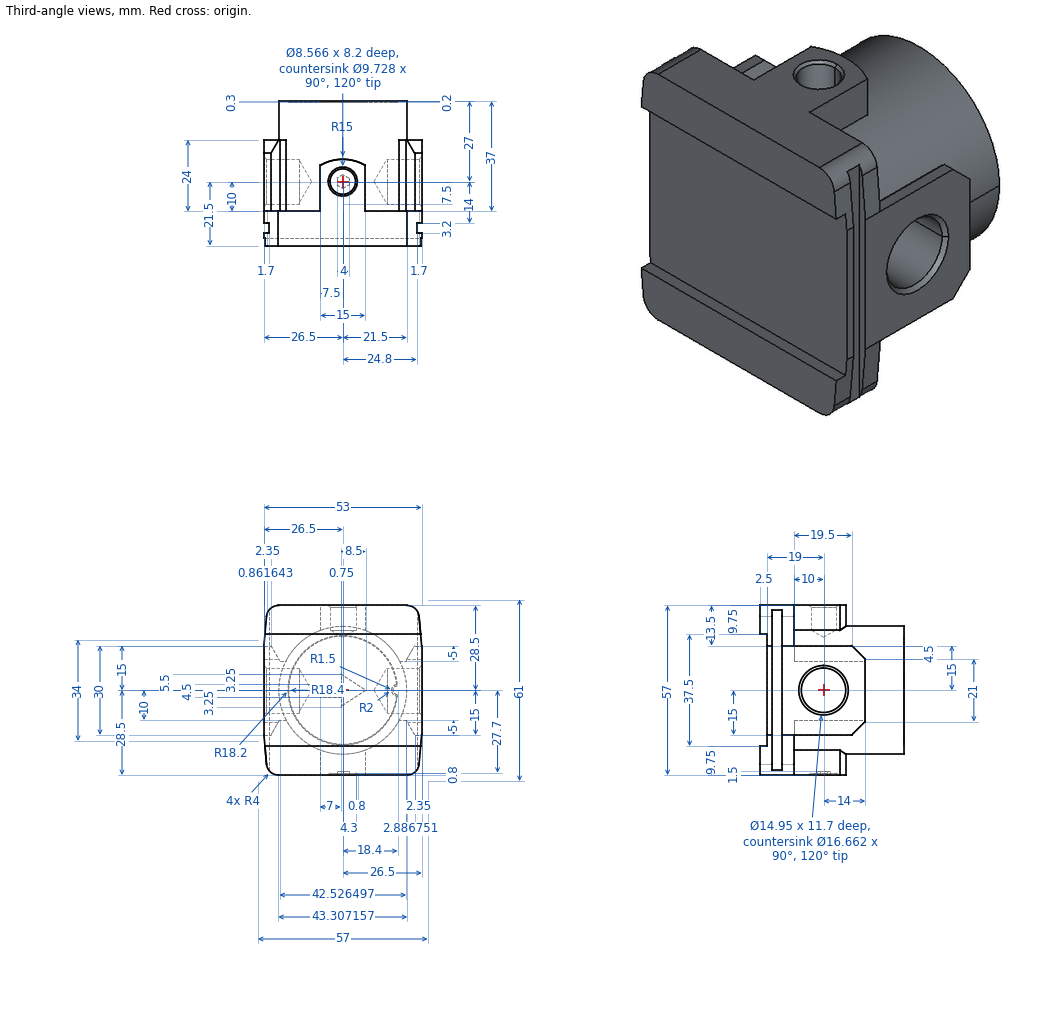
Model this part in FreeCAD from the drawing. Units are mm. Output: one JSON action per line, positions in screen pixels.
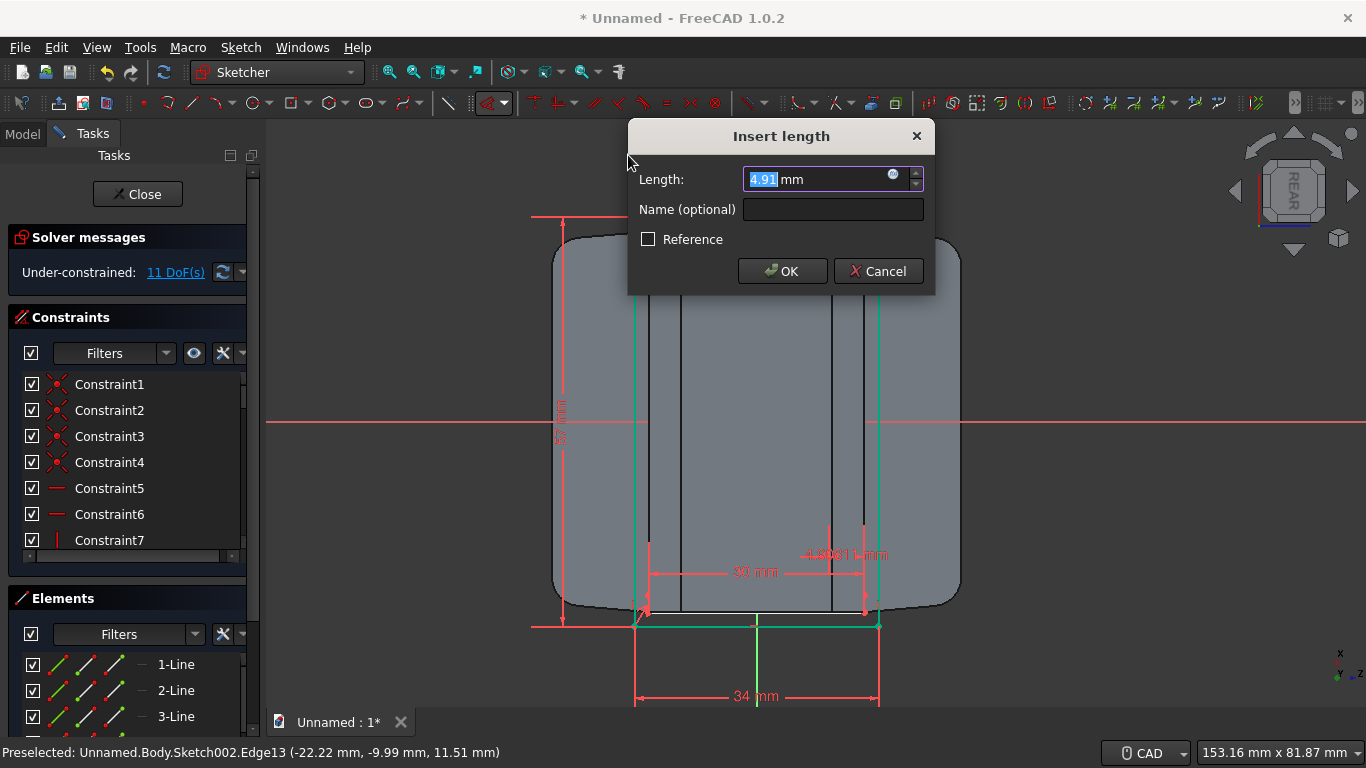
{"action": "type", "text": "5"}
{"action": "key", "text": "Return"}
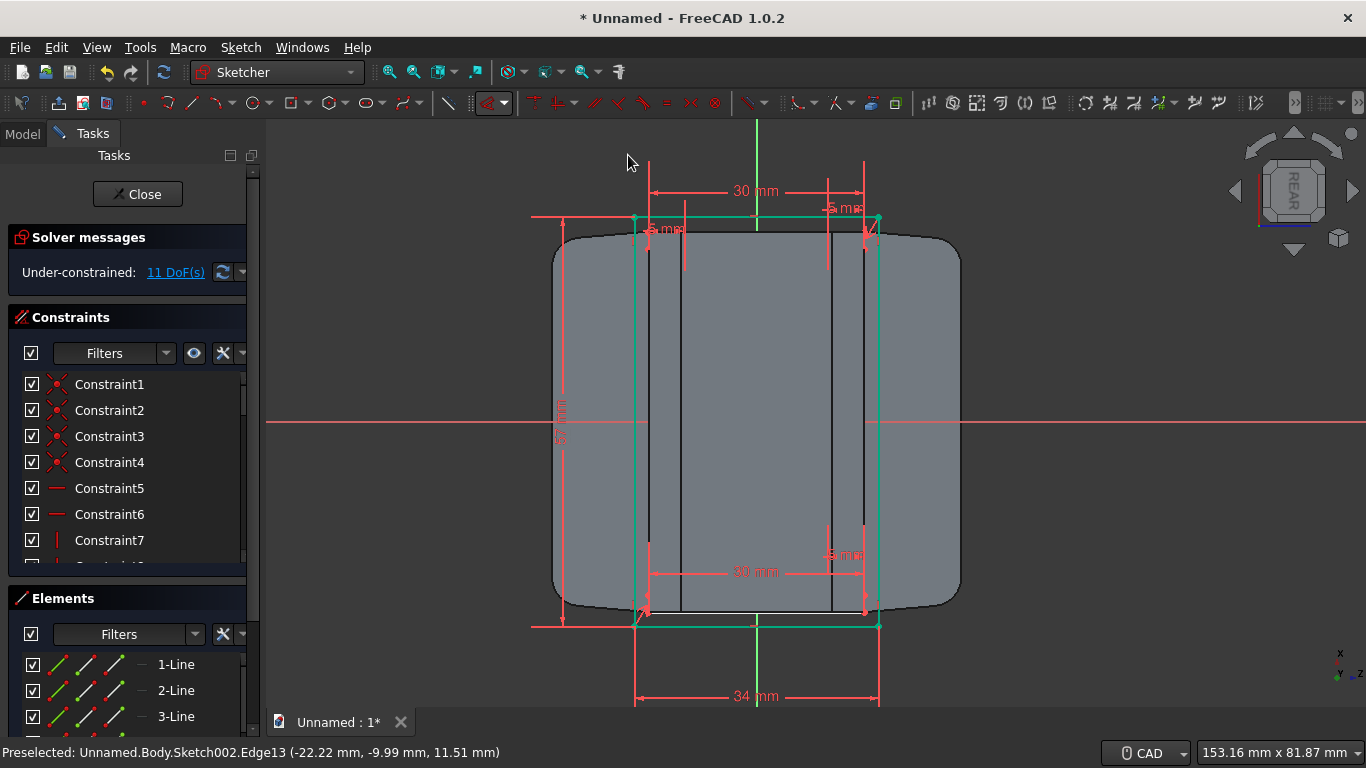
{"action": "left_click", "coordinate": [685, 576]}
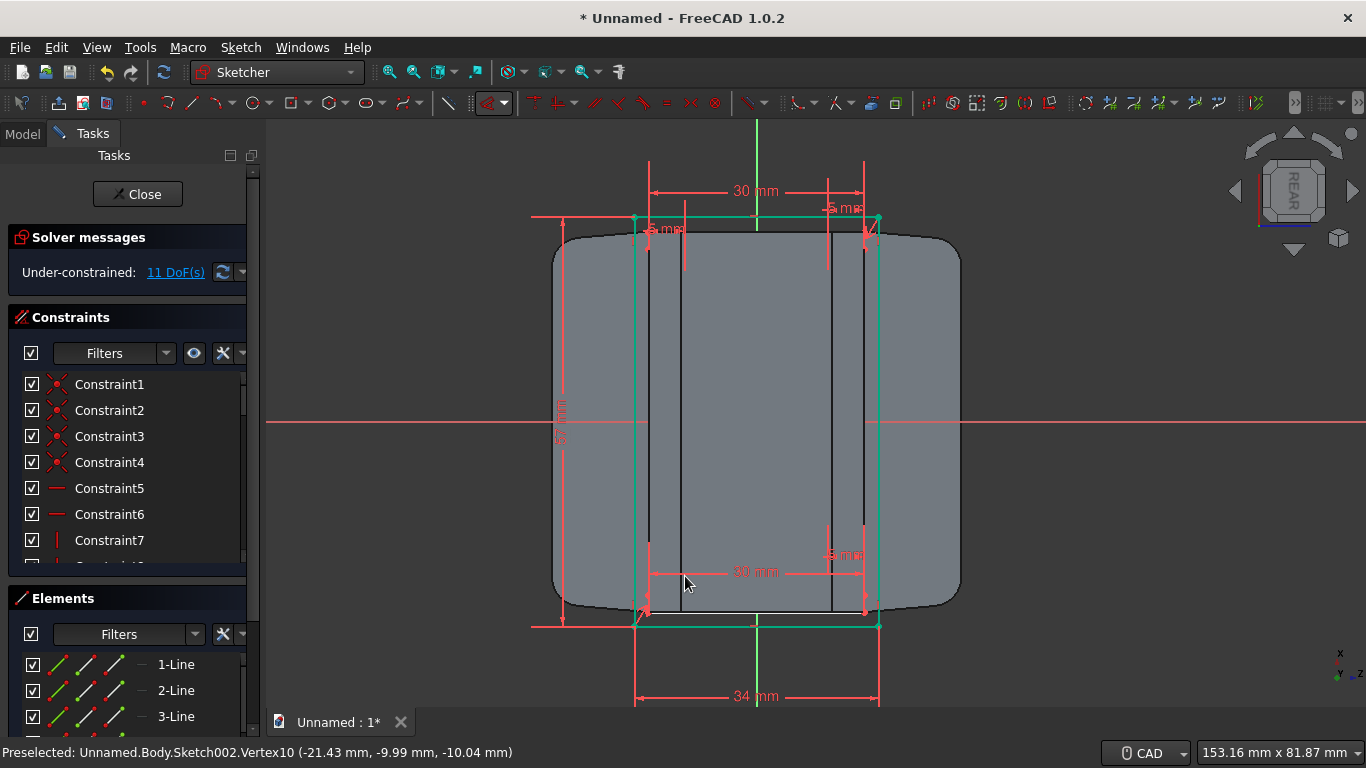
{"action": "left_click", "coordinate": [506, 104]}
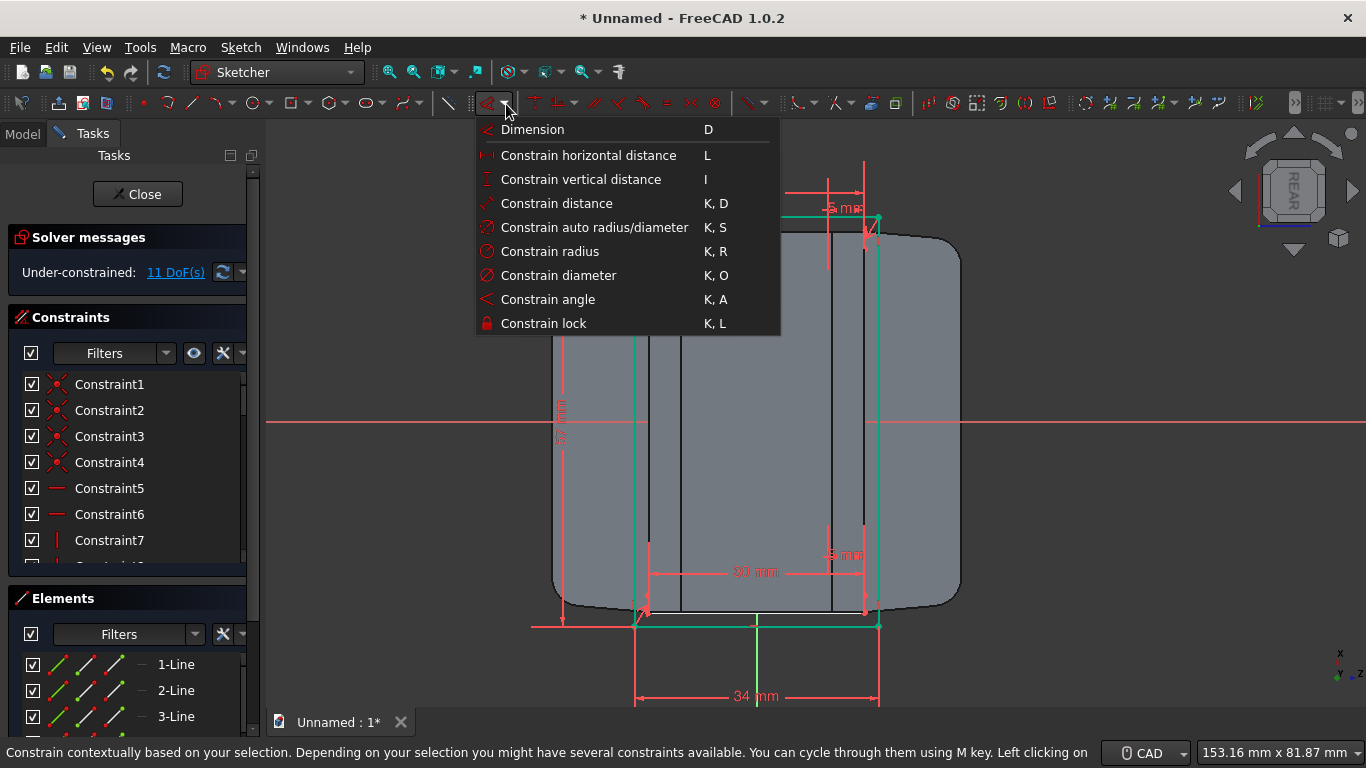
{"action": "left_click", "coordinate": [628, 155]}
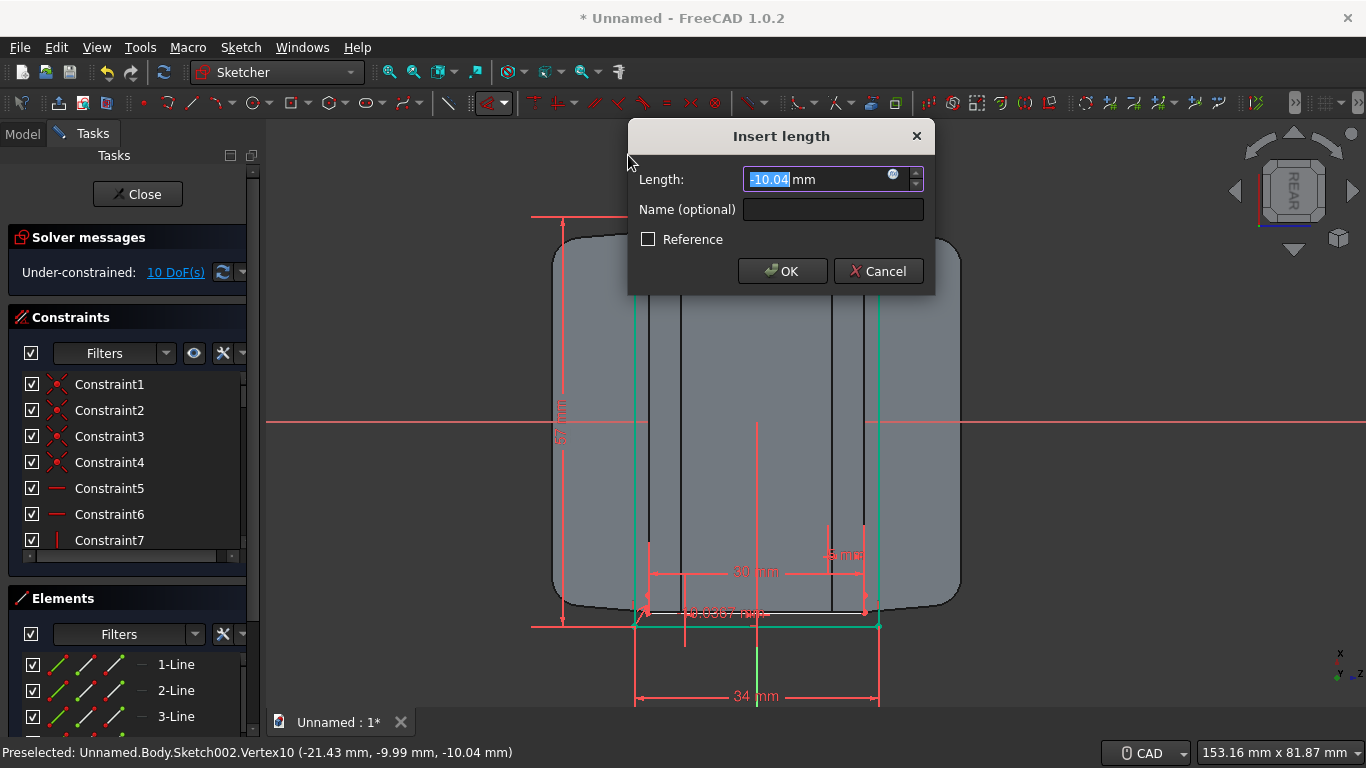
{"action": "type", "text": "-10"}
{"action": "key", "text": "Return"}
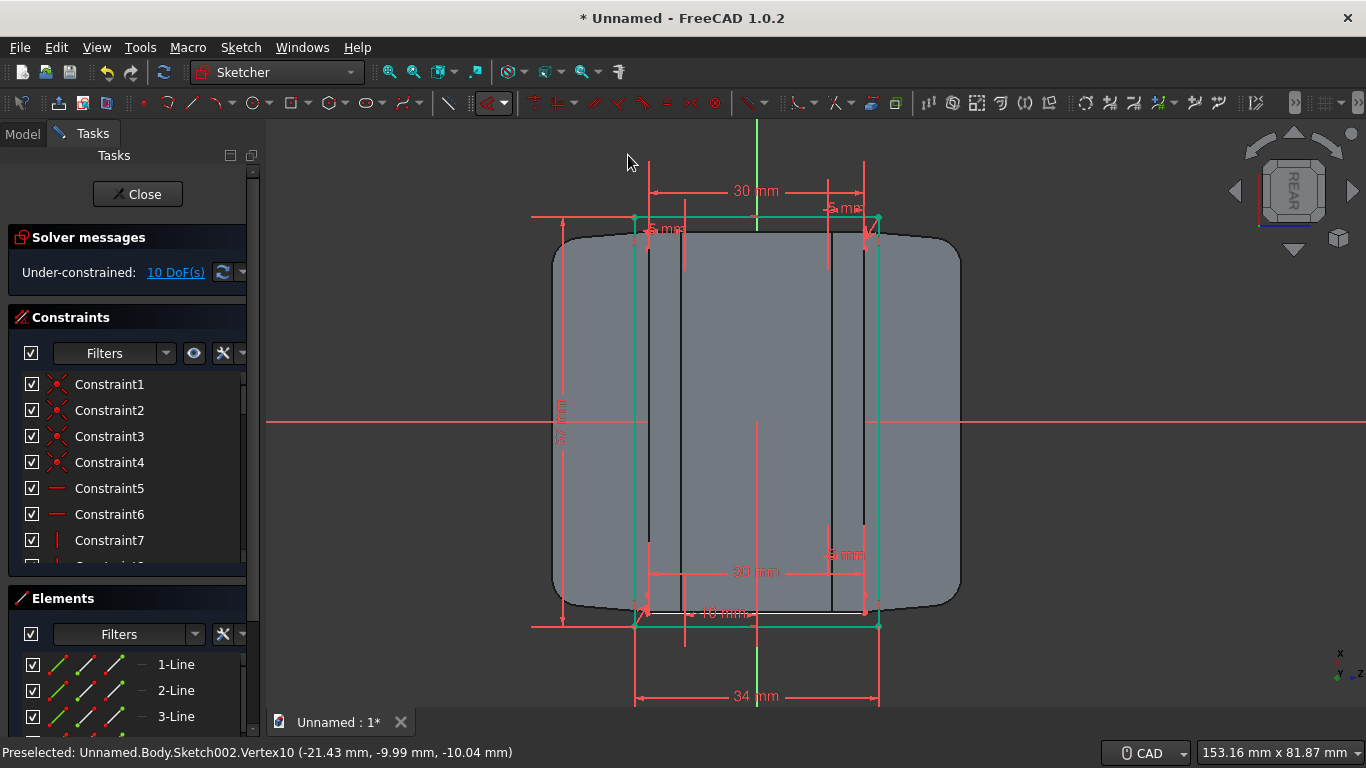
{"action": "scroll", "coordinate": [649, 241], "scroll_direction": "up", "scroll_amount": 5}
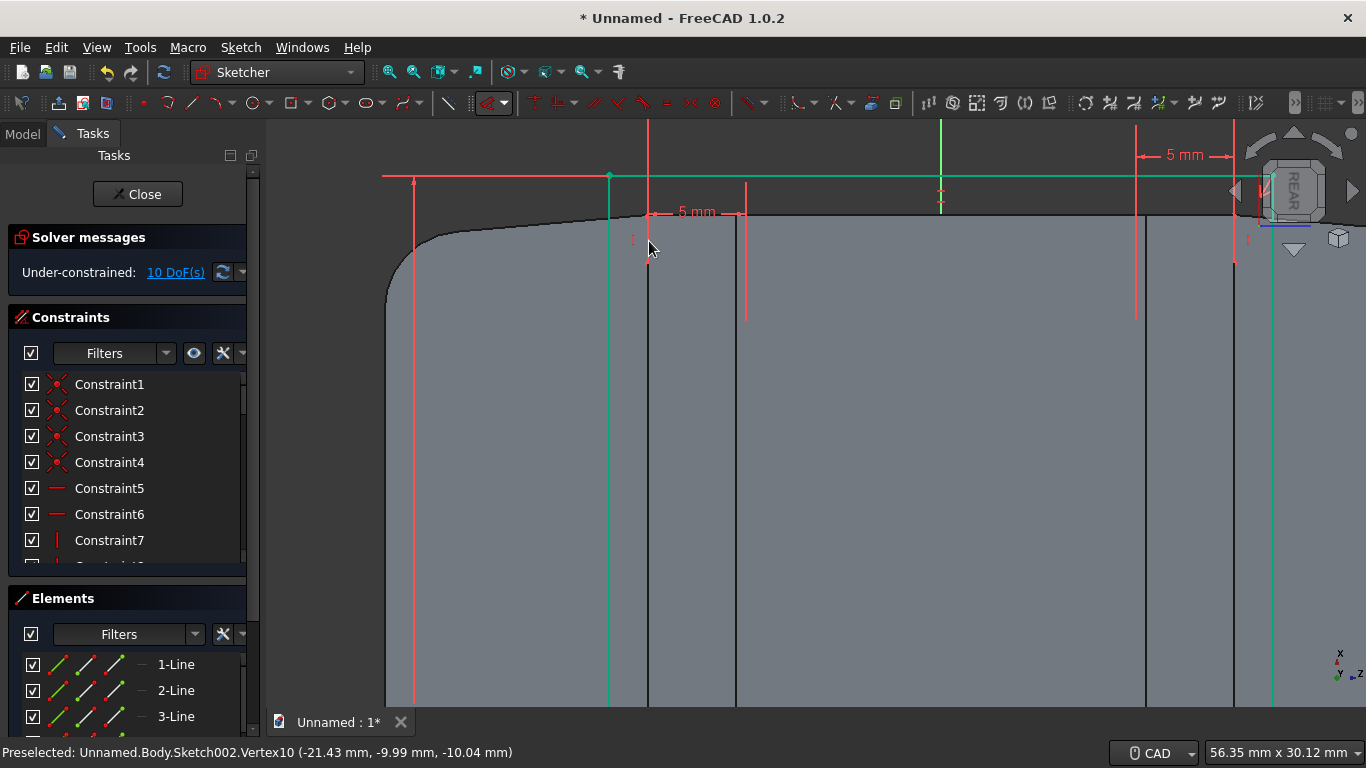
{"action": "left_click", "coordinate": [648, 240]}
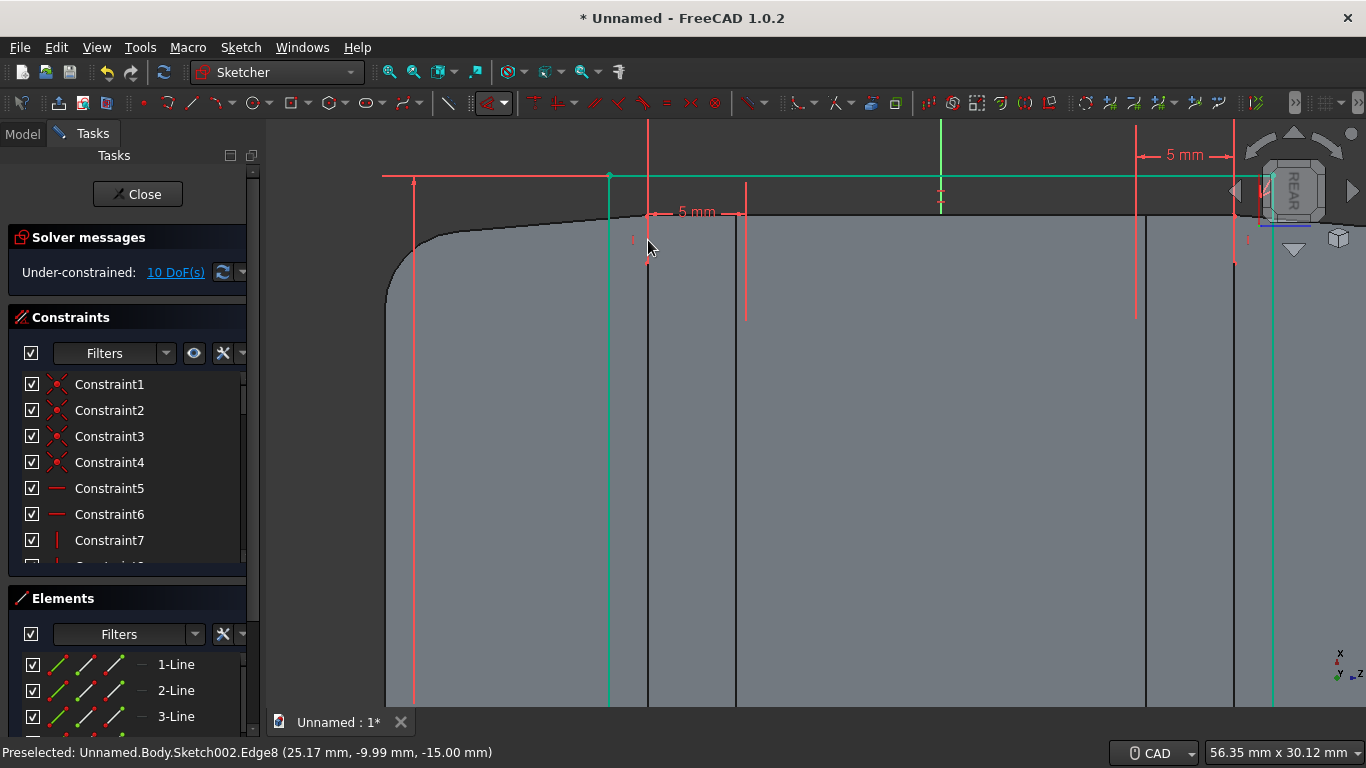
{"action": "left_click", "coordinate": [506, 104]}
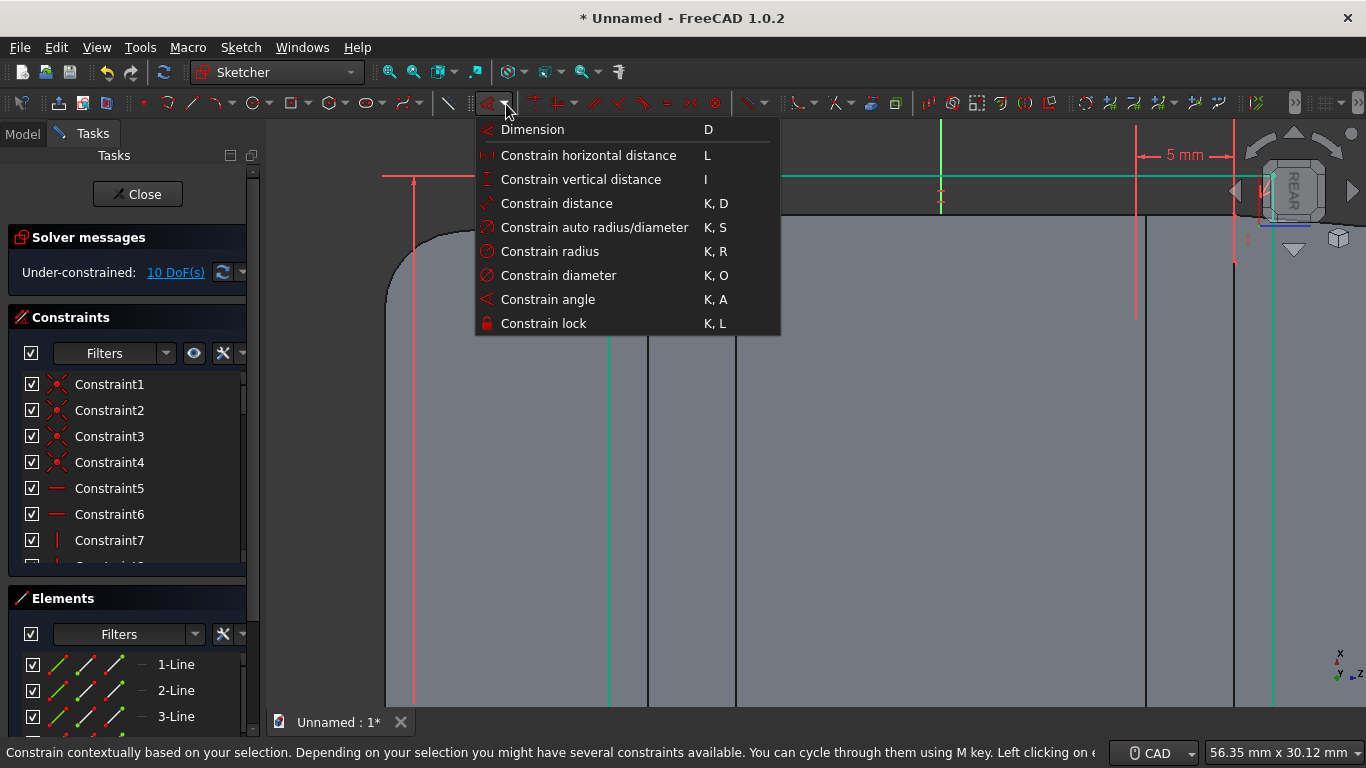
{"action": "left_click", "coordinate": [628, 179]}